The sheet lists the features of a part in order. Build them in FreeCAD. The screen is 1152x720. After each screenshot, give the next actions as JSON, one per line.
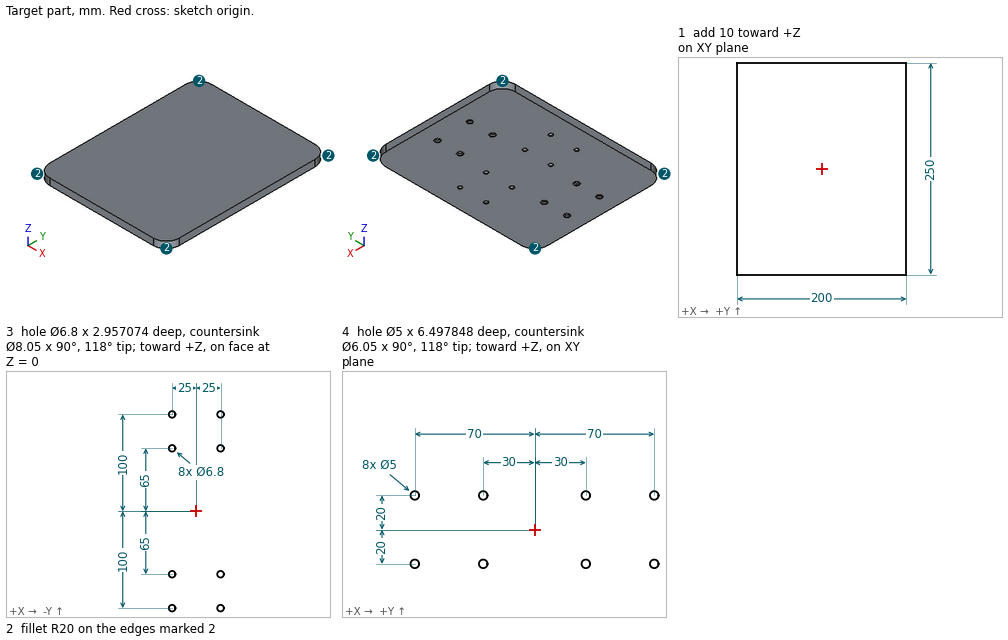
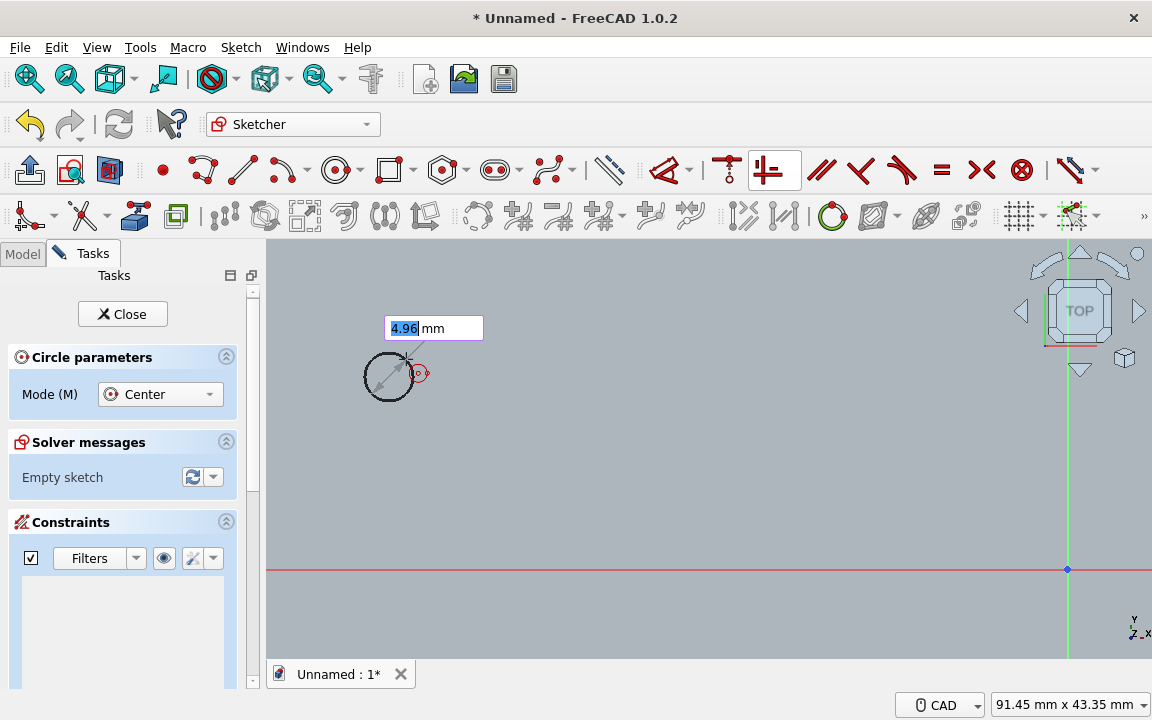
{"action": "type", "text": "5"}
{"action": "key", "text": "Return"}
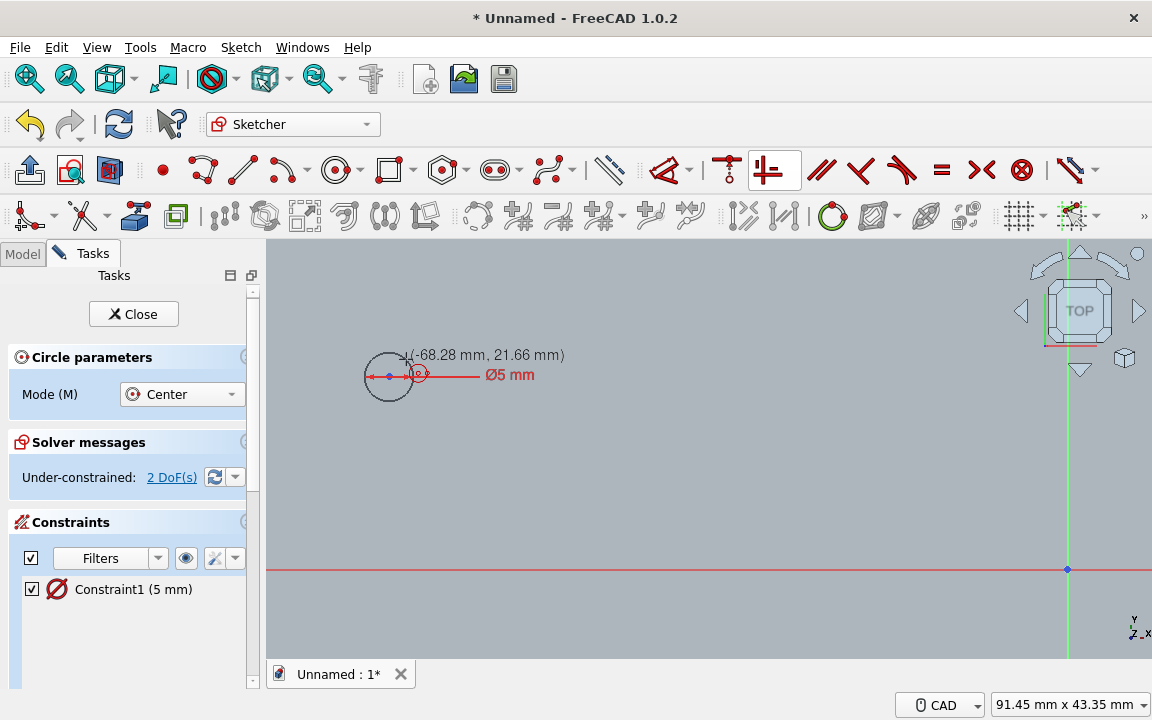
{"action": "left_click", "coordinate": [777, 376]}
{"action": "mouse_move", "coordinate": [794, 359]}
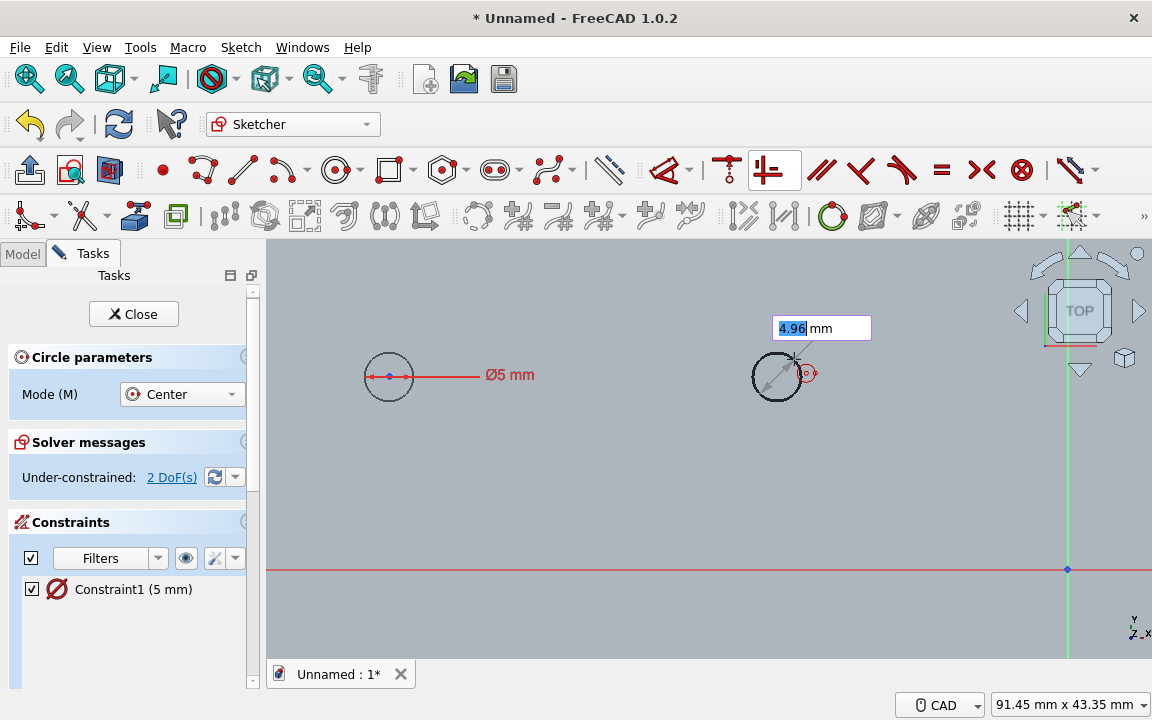
{"action": "type", "text": "5"}
{"action": "key", "text": "Return"}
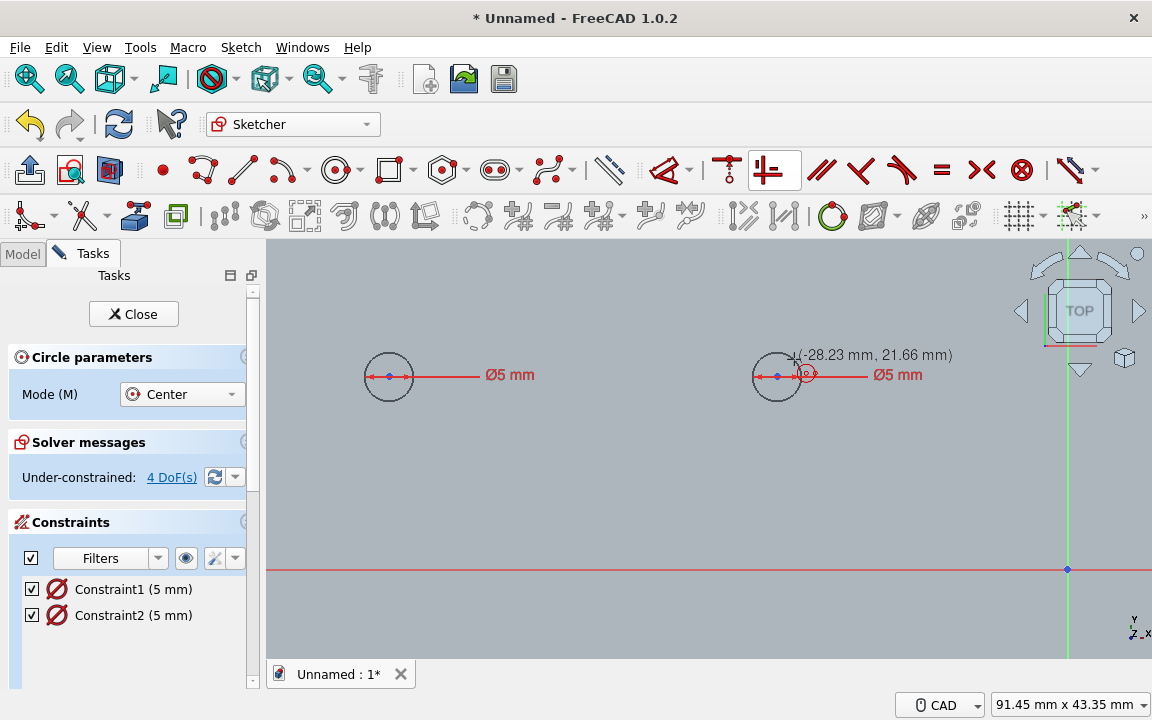
{"action": "scroll", "coordinate": [392, 379], "scroll_direction": "down", "scroll_amount": 5}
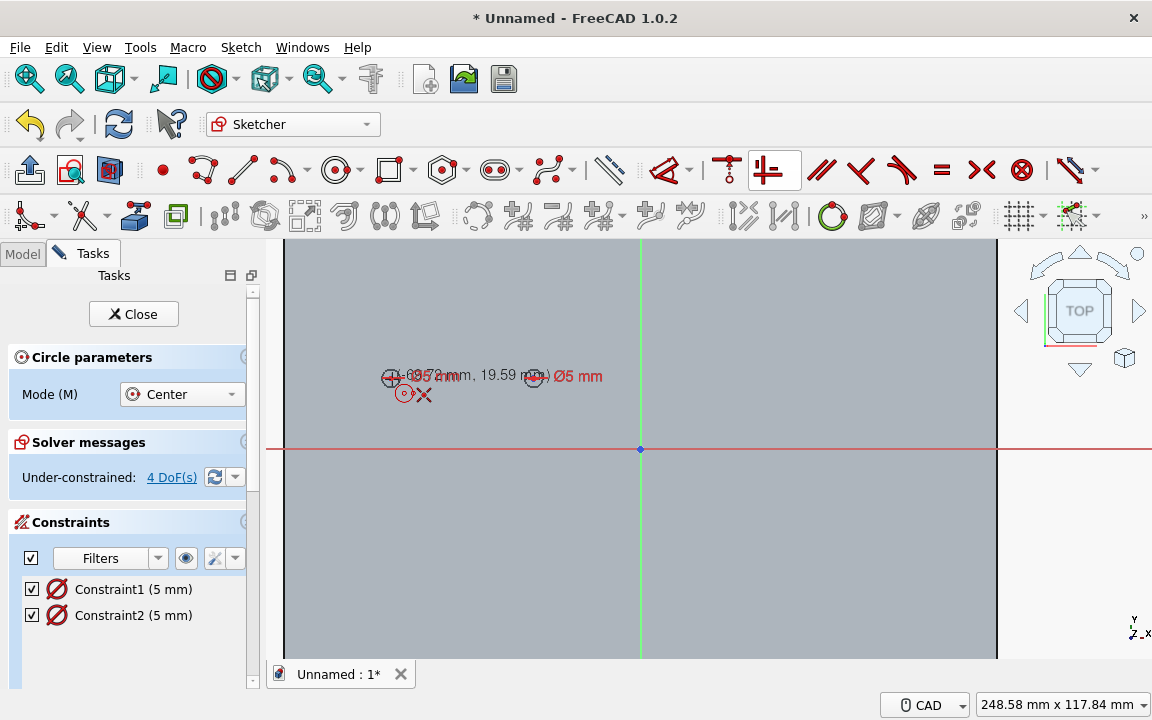
{"action": "scroll", "coordinate": [391, 521], "scroll_direction": "up", "scroll_amount": 5}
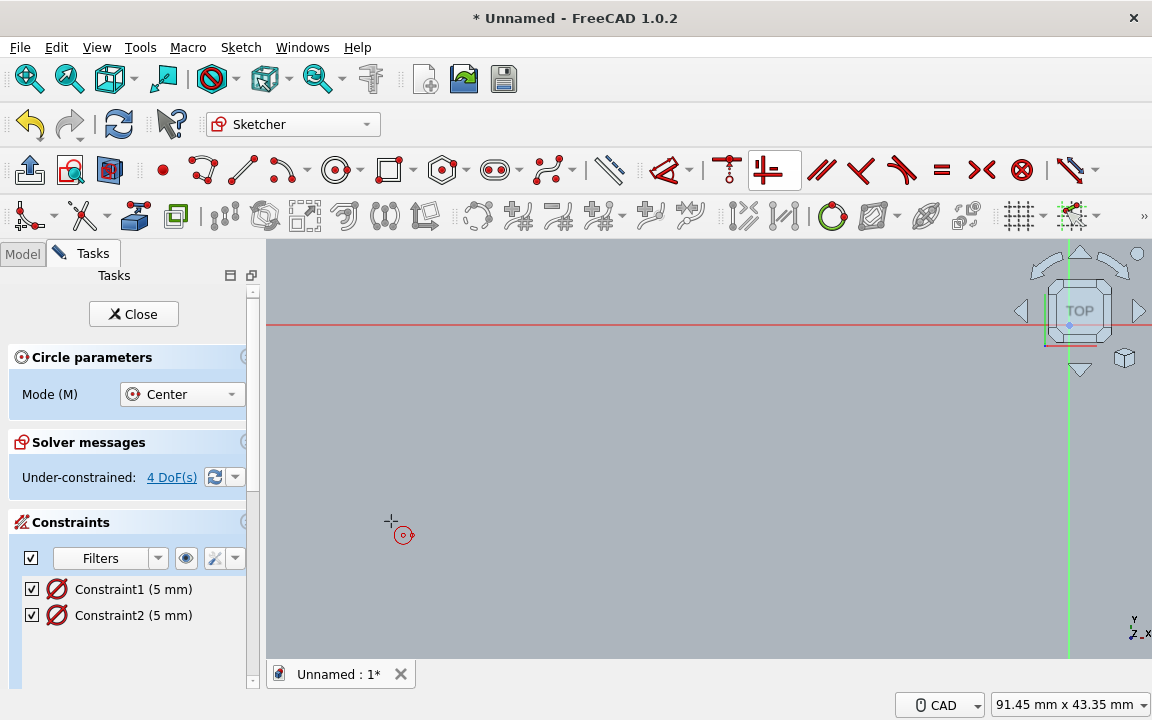
{"action": "left_click", "coordinate": [391, 519]}
{"action": "mouse_move", "coordinate": [408, 502]}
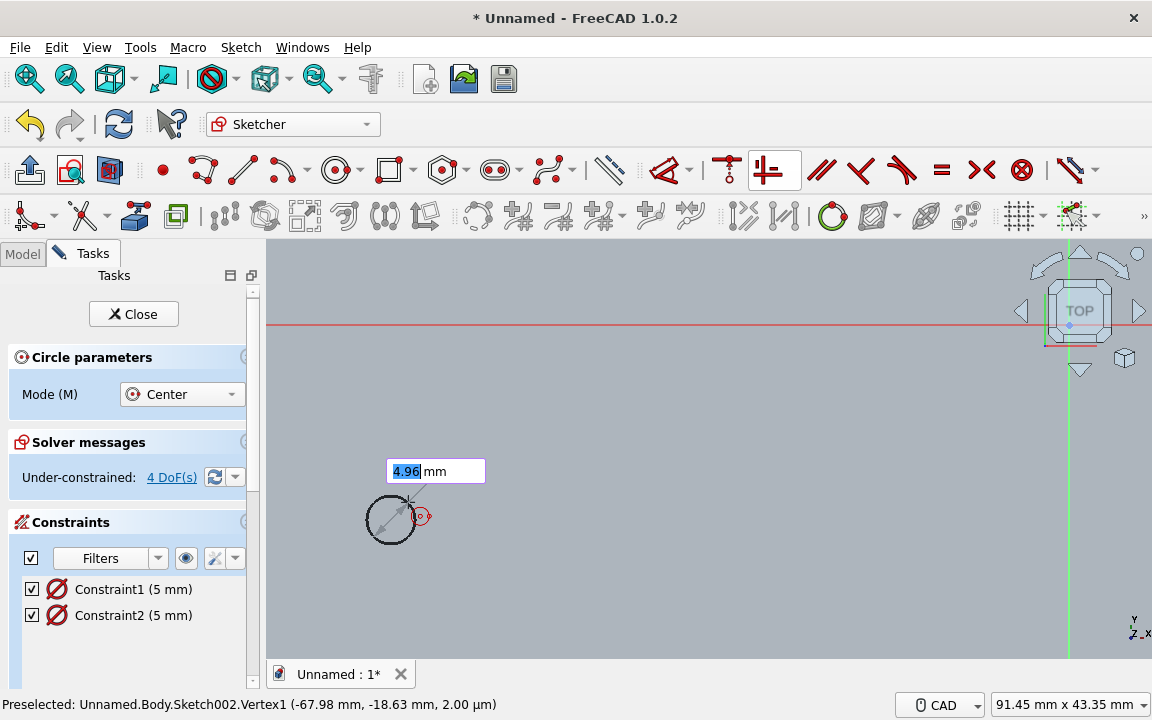
{"action": "type", "text": "5"}
{"action": "key", "text": "Return"}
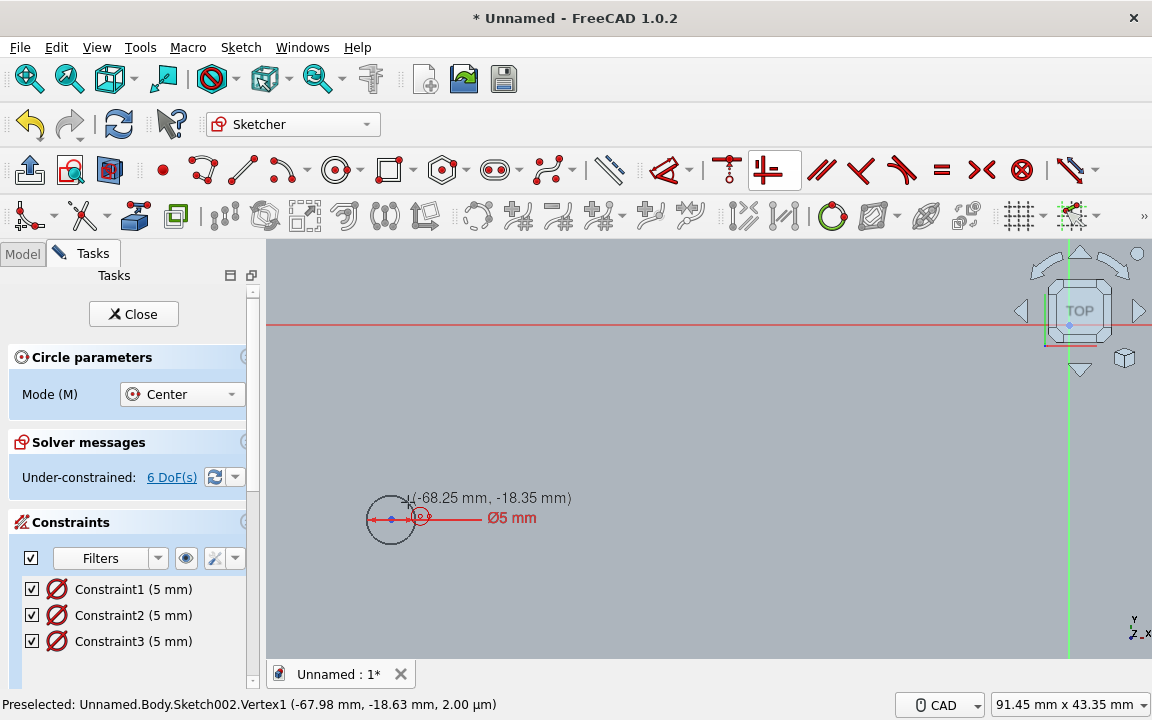
{"action": "left_click", "coordinate": [779, 519]}
{"action": "mouse_move", "coordinate": [796, 502]}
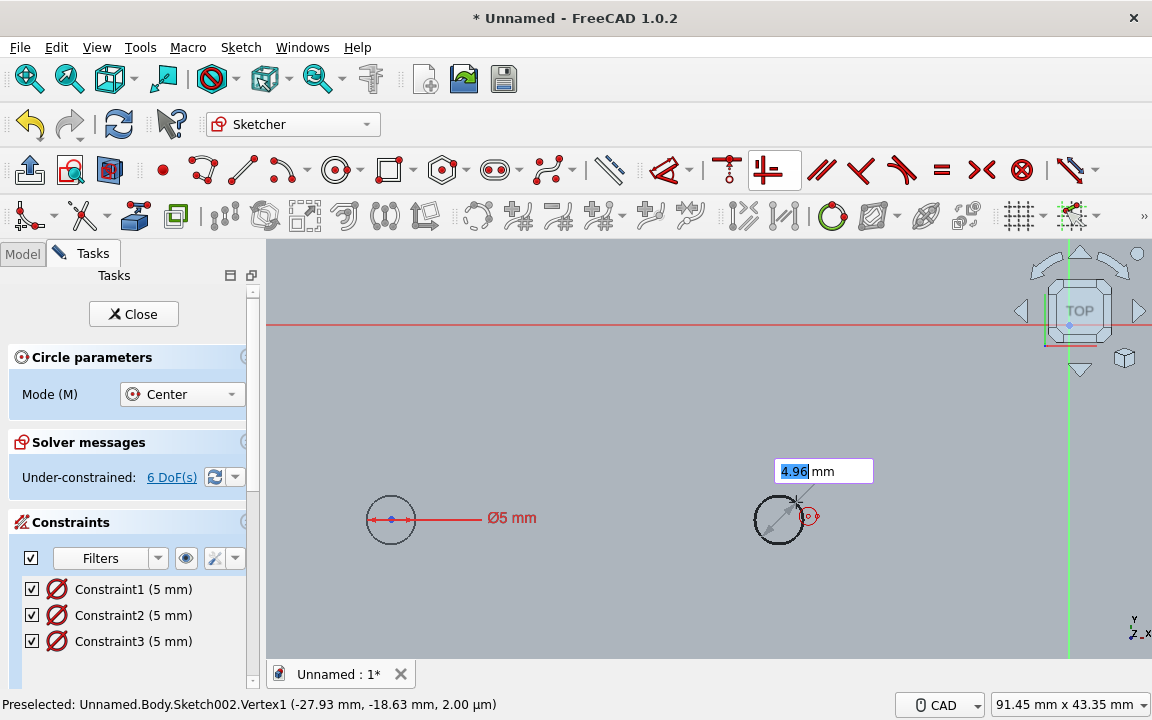
{"action": "type", "text": "5"}
{"action": "key", "text": "Return"}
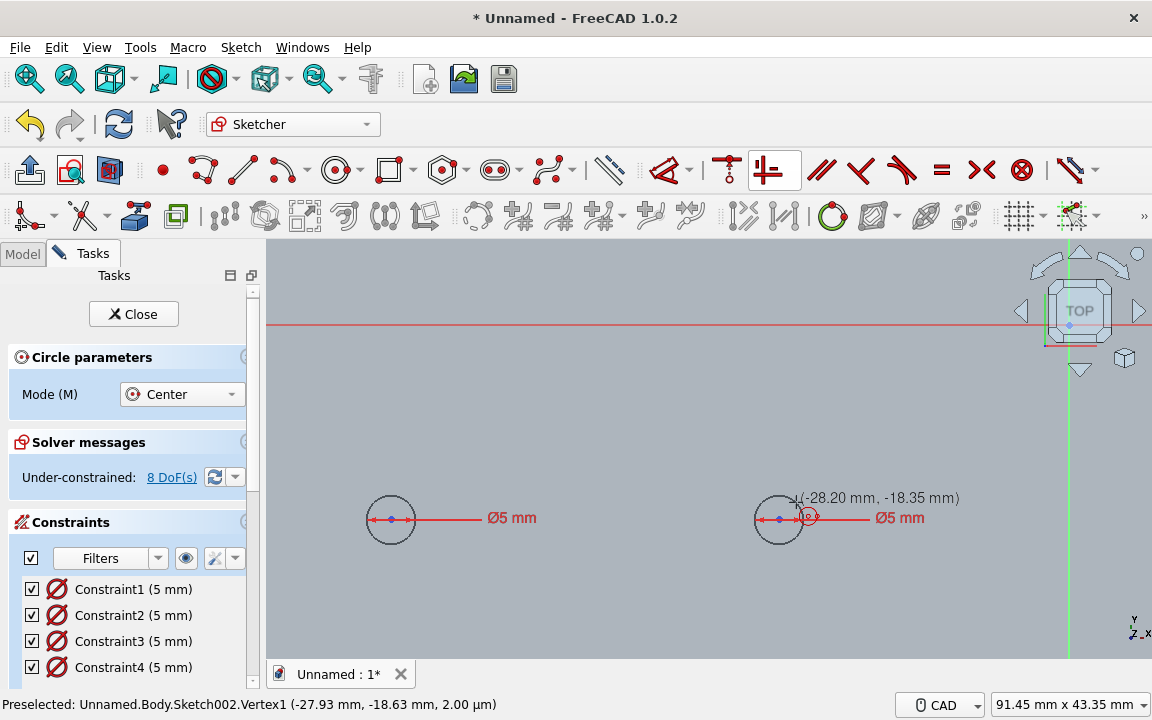
{"action": "scroll", "coordinate": [391, 521], "scroll_direction": "down", "scroll_amount": 5}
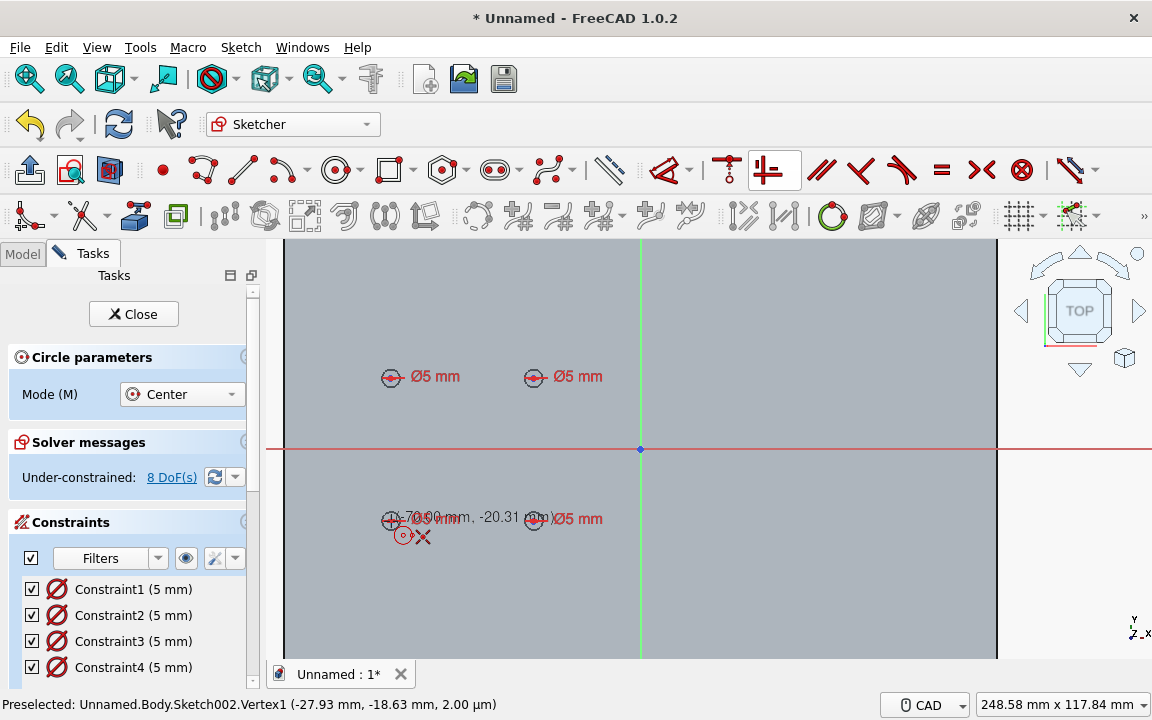
{"action": "scroll", "coordinate": [748, 378], "scroll_direction": "up", "scroll_amount": 5}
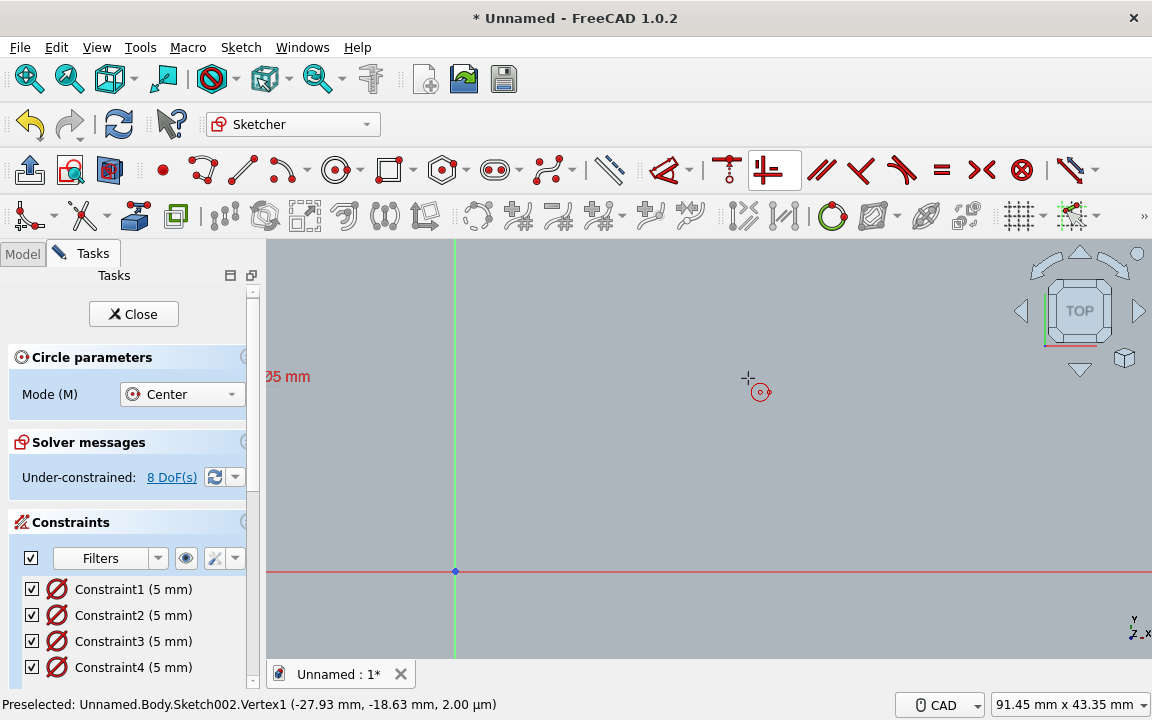
{"action": "left_click", "coordinate": [746, 378]}
{"action": "mouse_move", "coordinate": [763, 361]}